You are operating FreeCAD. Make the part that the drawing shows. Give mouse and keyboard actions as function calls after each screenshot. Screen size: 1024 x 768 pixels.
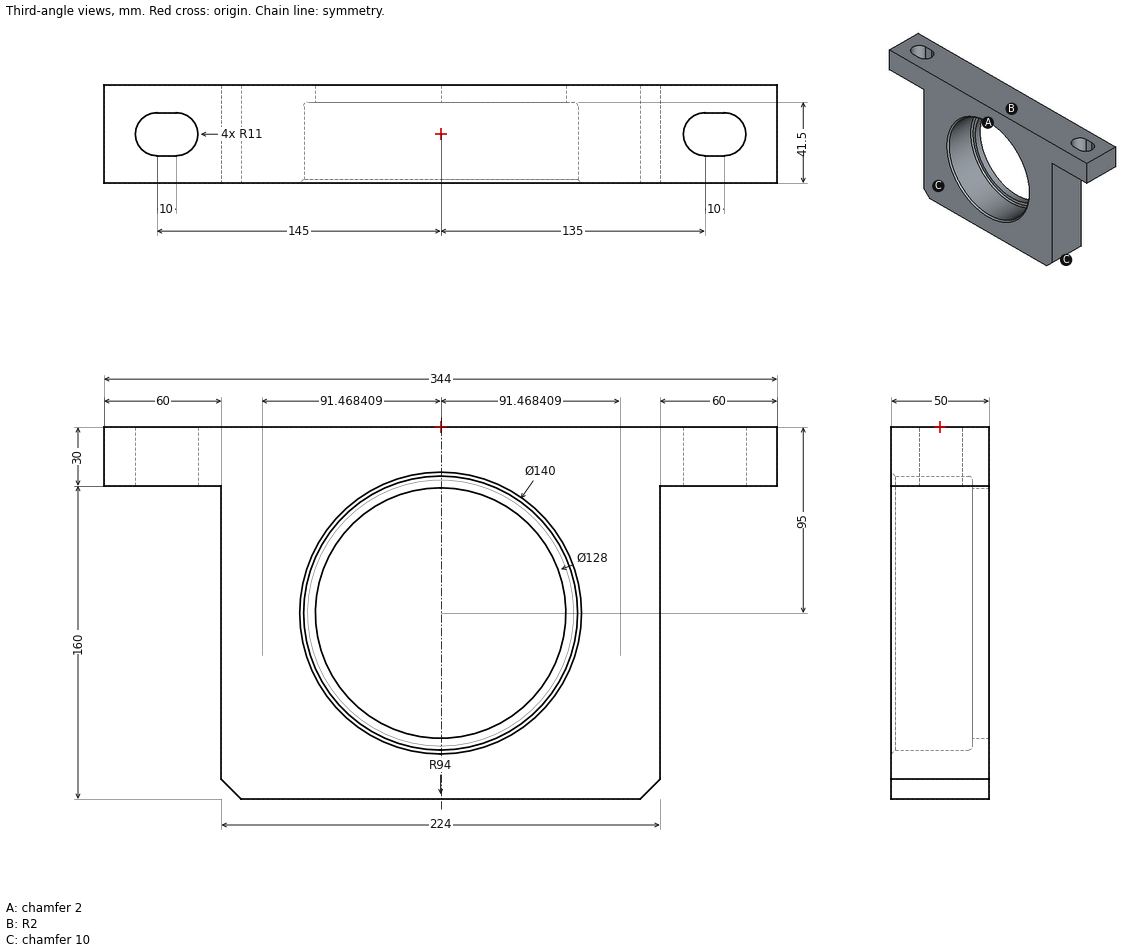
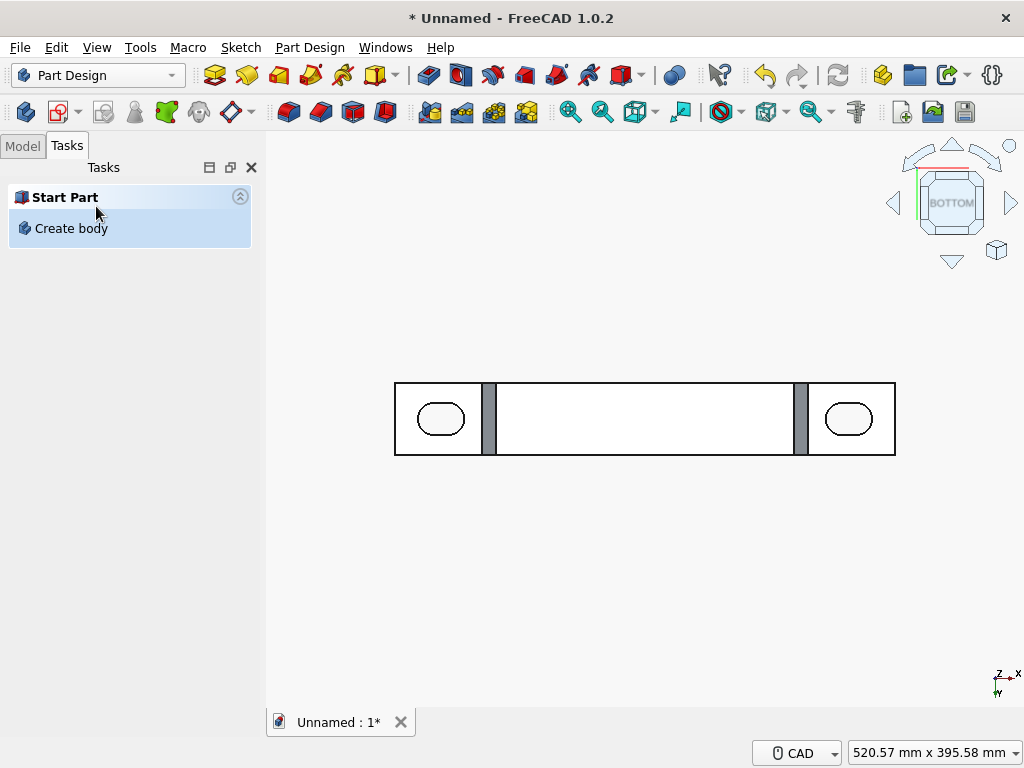
key(0)